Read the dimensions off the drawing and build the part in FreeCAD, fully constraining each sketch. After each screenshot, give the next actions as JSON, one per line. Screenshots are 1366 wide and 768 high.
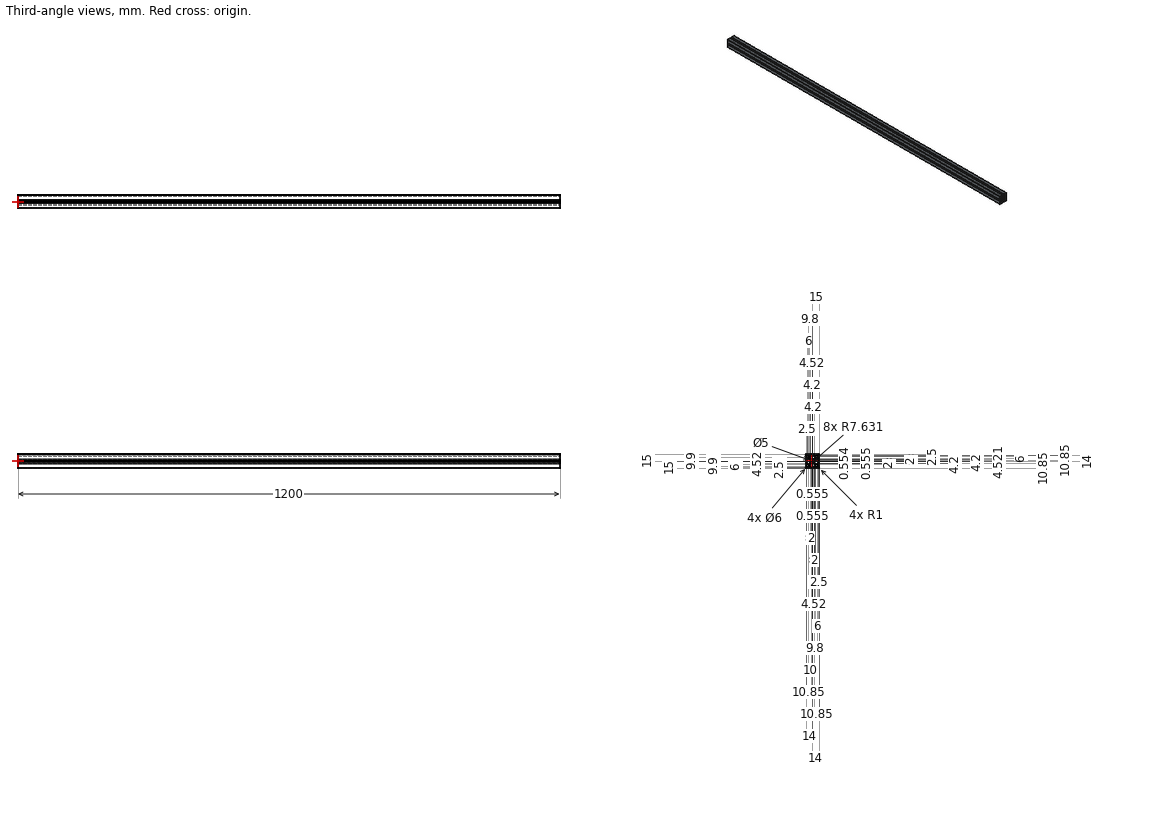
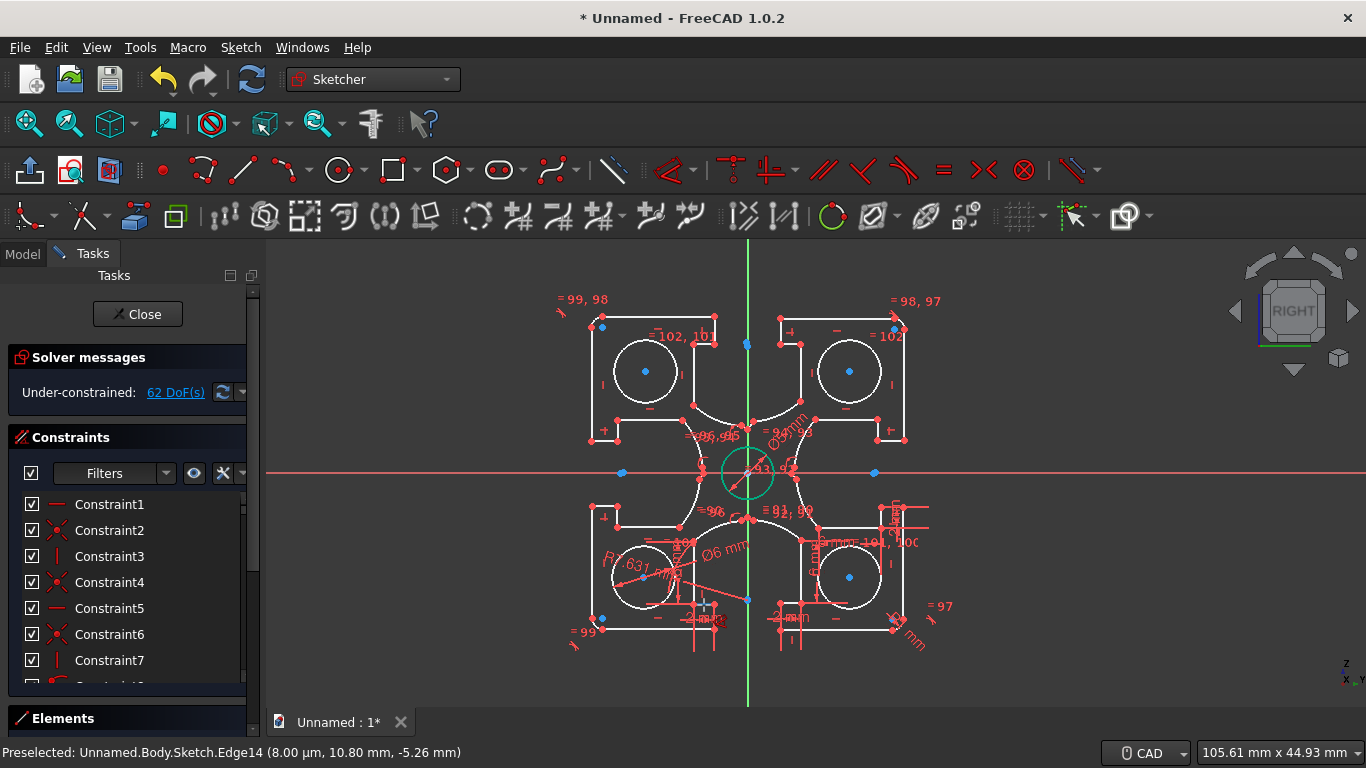
{"action": "left_click", "coordinate": [834, 420]}
{"action": "left_click", "coordinate": [846, 386]}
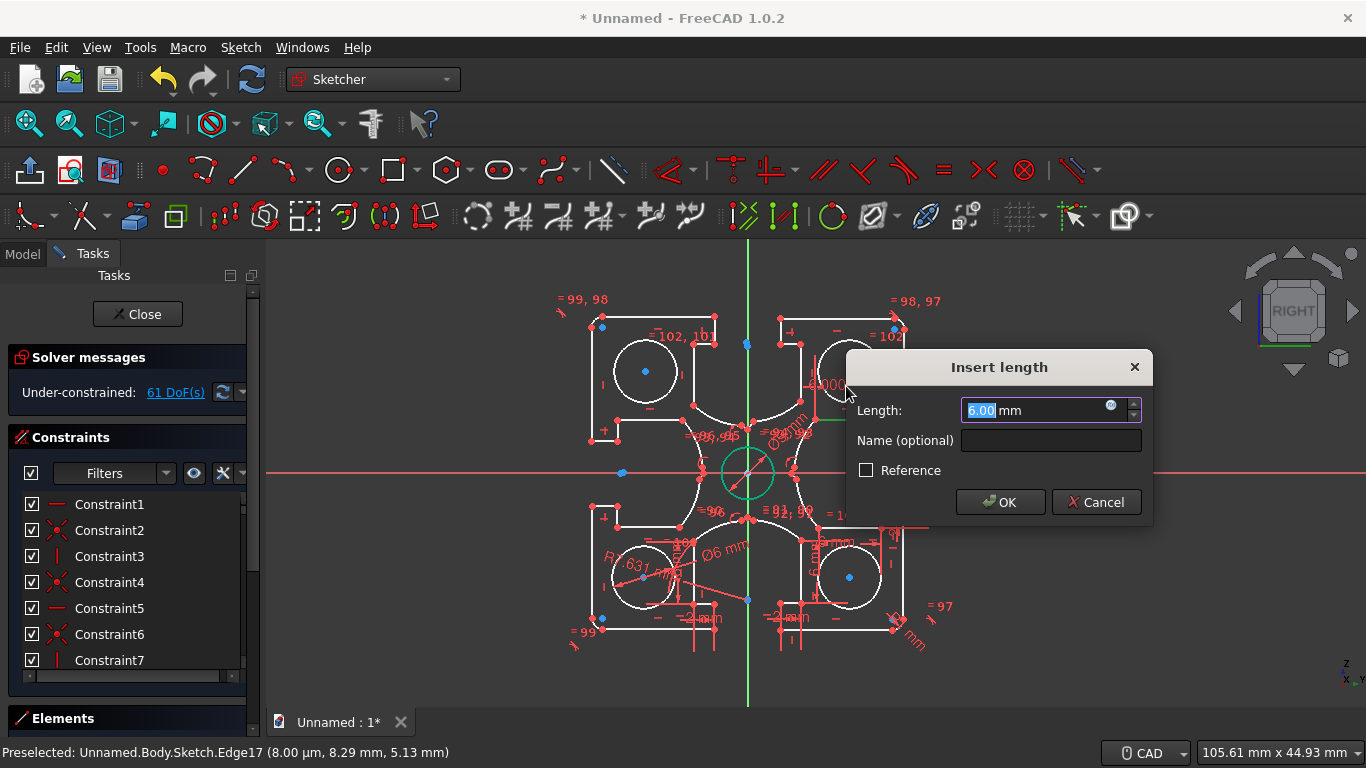
{"action": "type", "text": "6"}
{"action": "key", "text": "Return"}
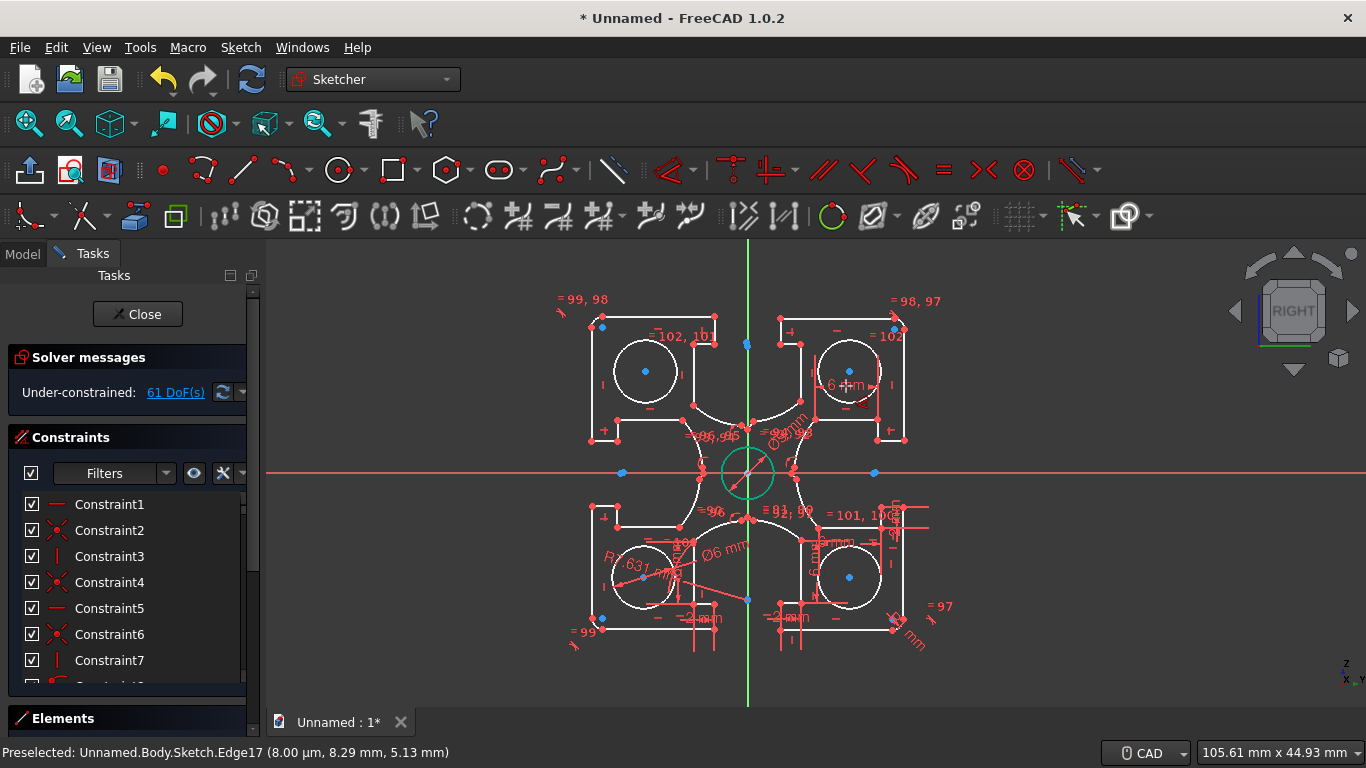
{"action": "scroll", "coordinate": [878, 430], "scroll_direction": "up", "scroll_amount": 4}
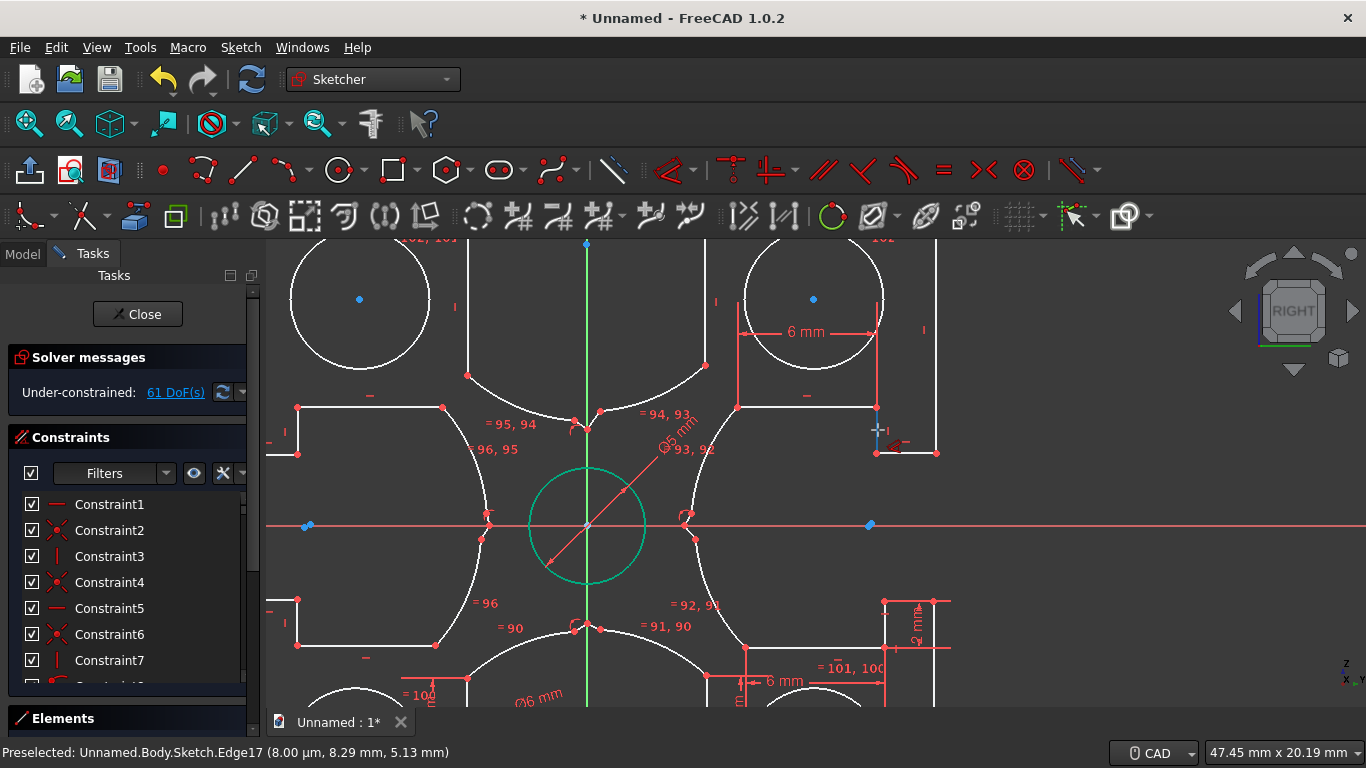
{"action": "left_click", "coordinate": [877, 430]}
{"action": "left_click", "coordinate": [911, 430]}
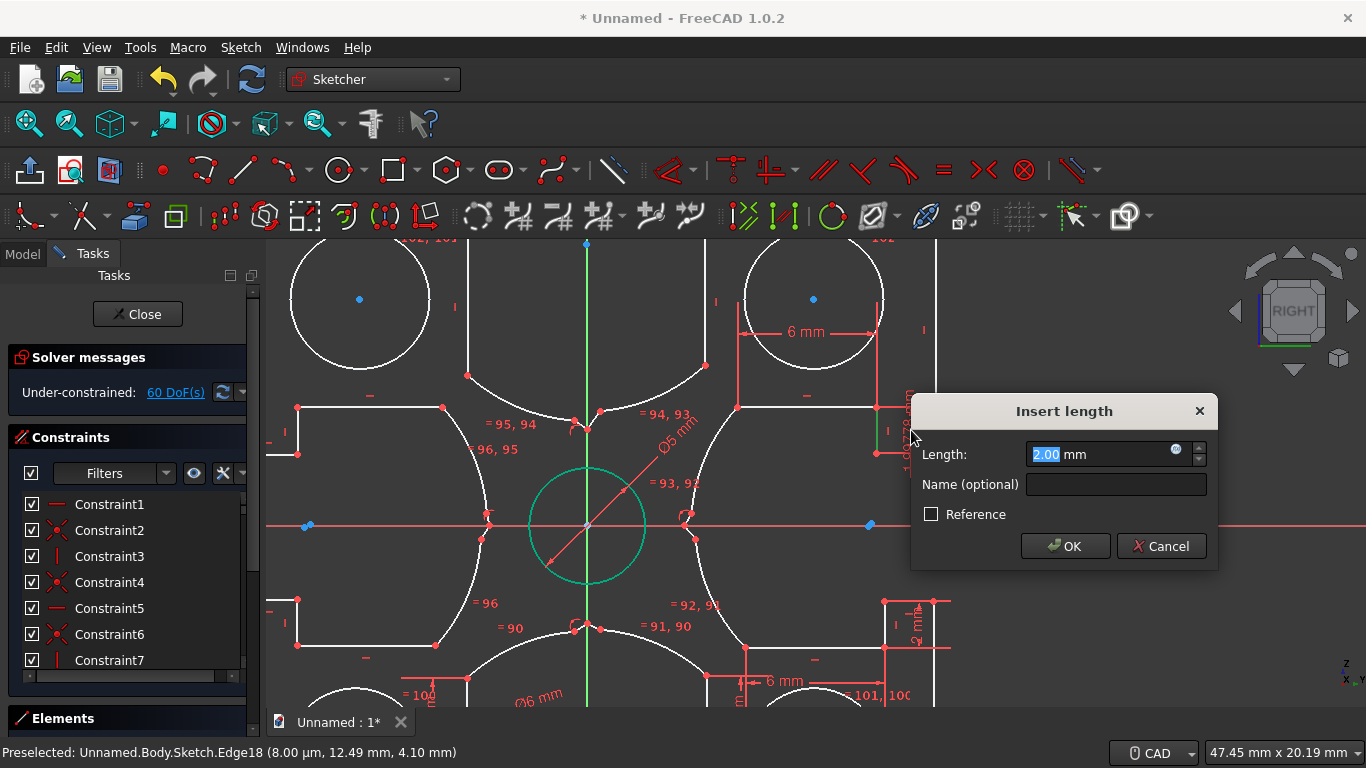
{"action": "type", "text": "2"}
{"action": "key", "text": "Return"}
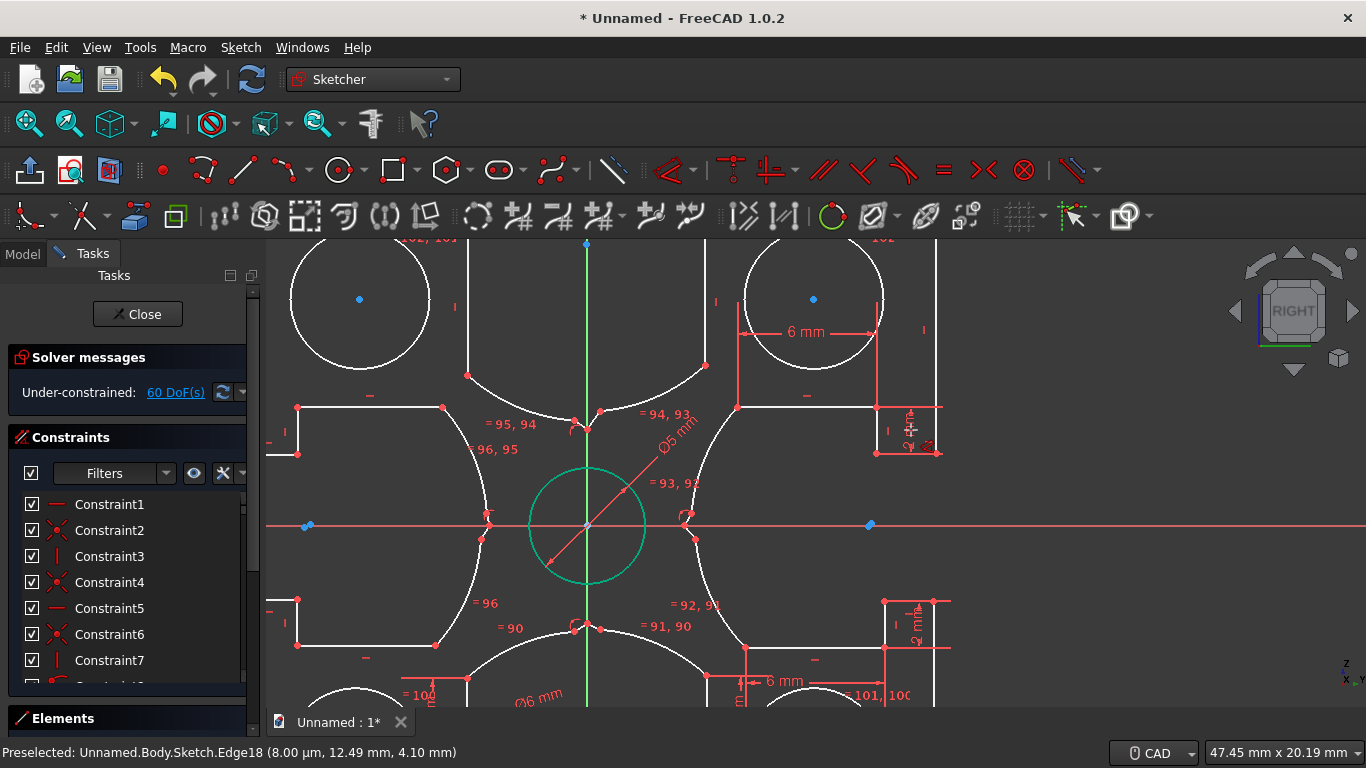
{"action": "scroll", "coordinate": [878, 430], "scroll_direction": "down", "scroll_amount": 4}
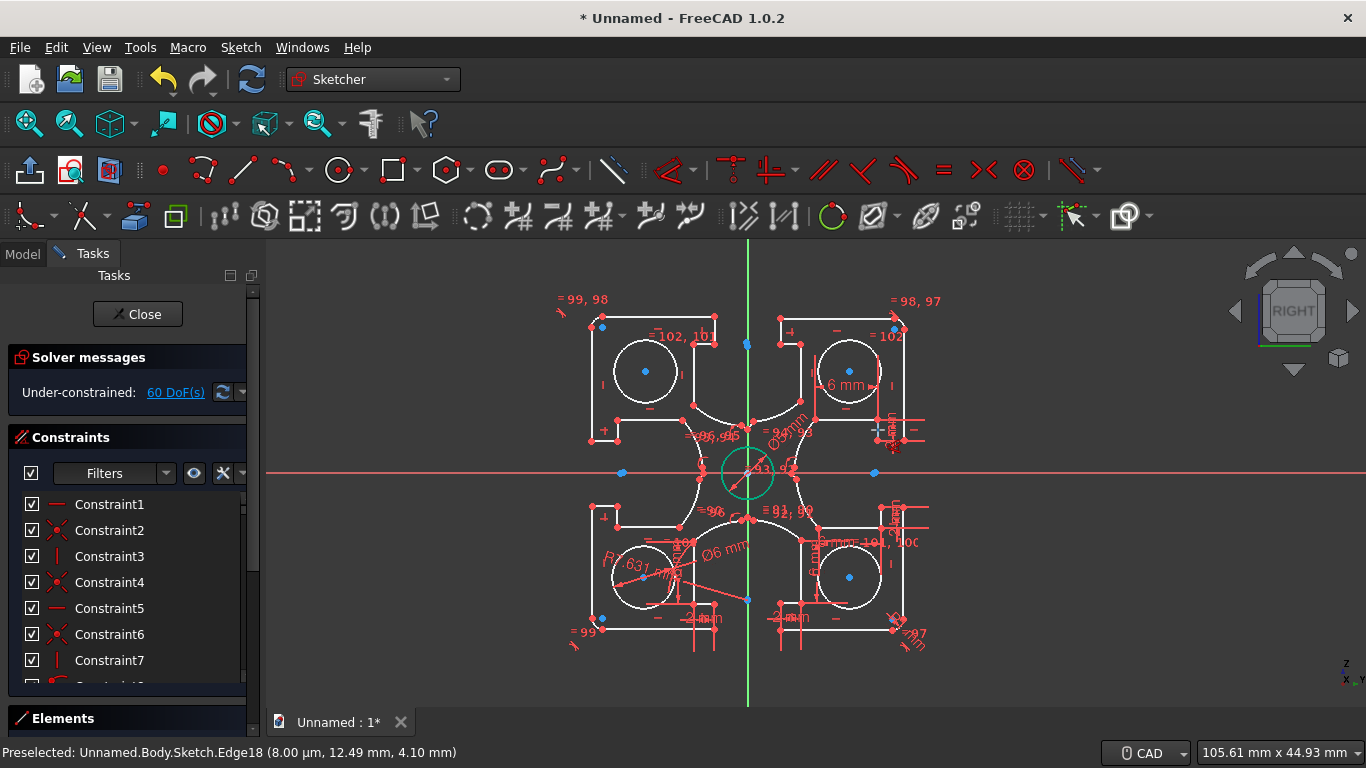
{"action": "scroll", "coordinate": [787, 344], "scroll_direction": "up", "scroll_amount": 5}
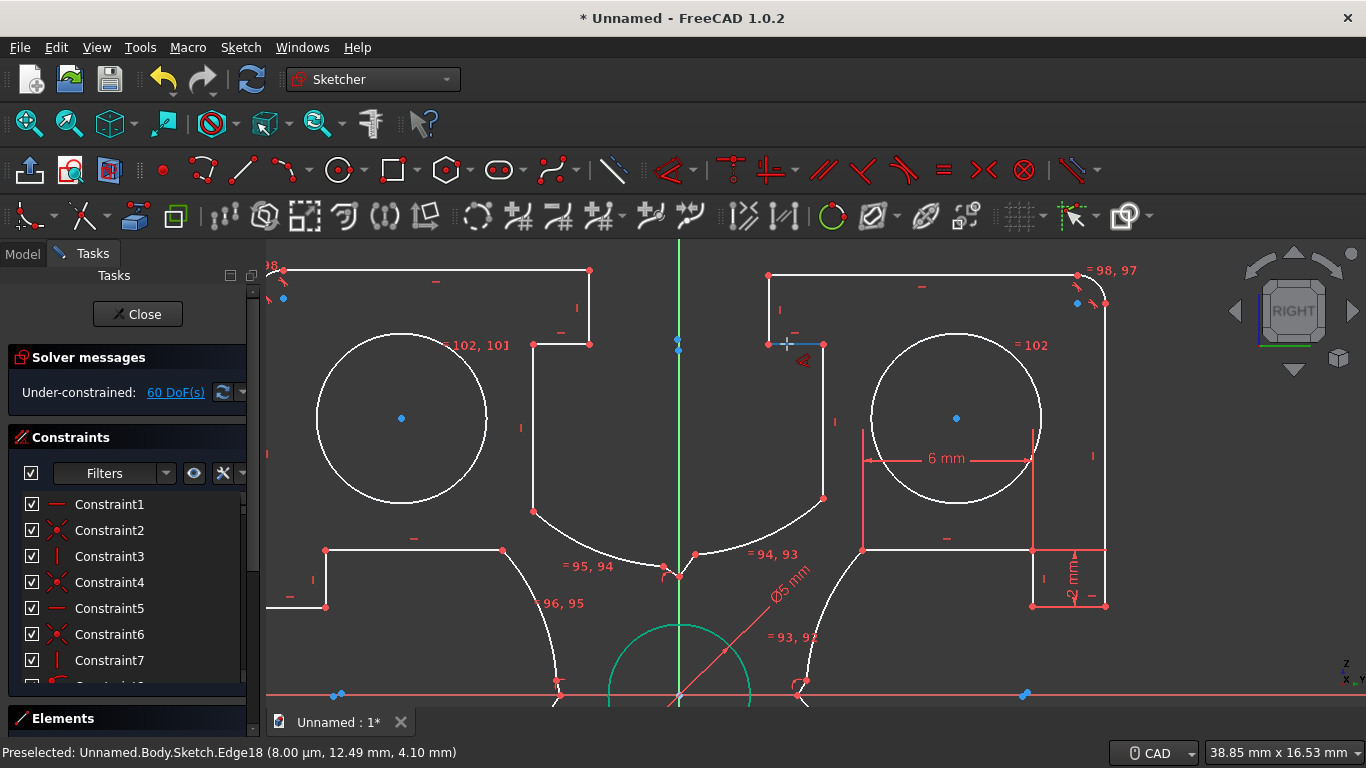
{"action": "left_click", "coordinate": [785, 344]}
{"action": "left_click", "coordinate": [796, 310]}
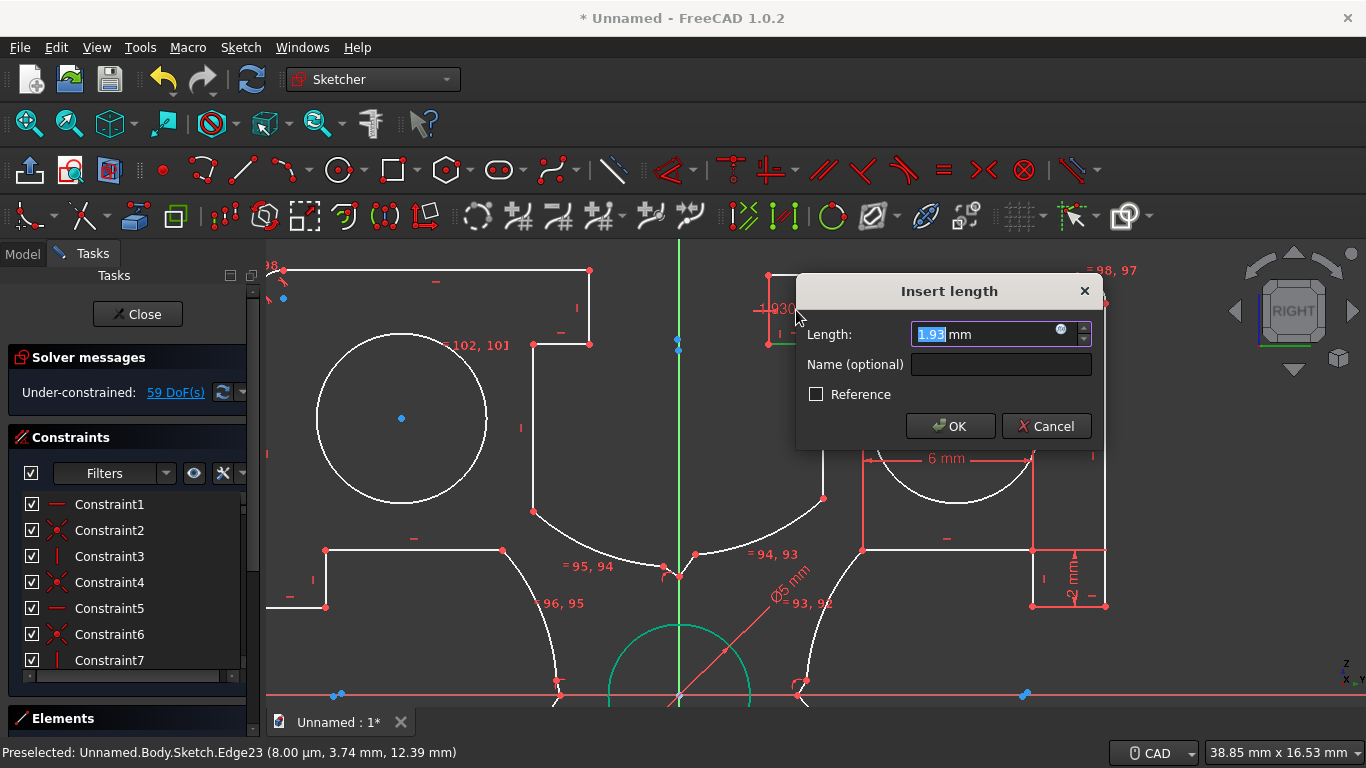
{"action": "type", "text": "2"}
{"action": "key", "text": "Return"}